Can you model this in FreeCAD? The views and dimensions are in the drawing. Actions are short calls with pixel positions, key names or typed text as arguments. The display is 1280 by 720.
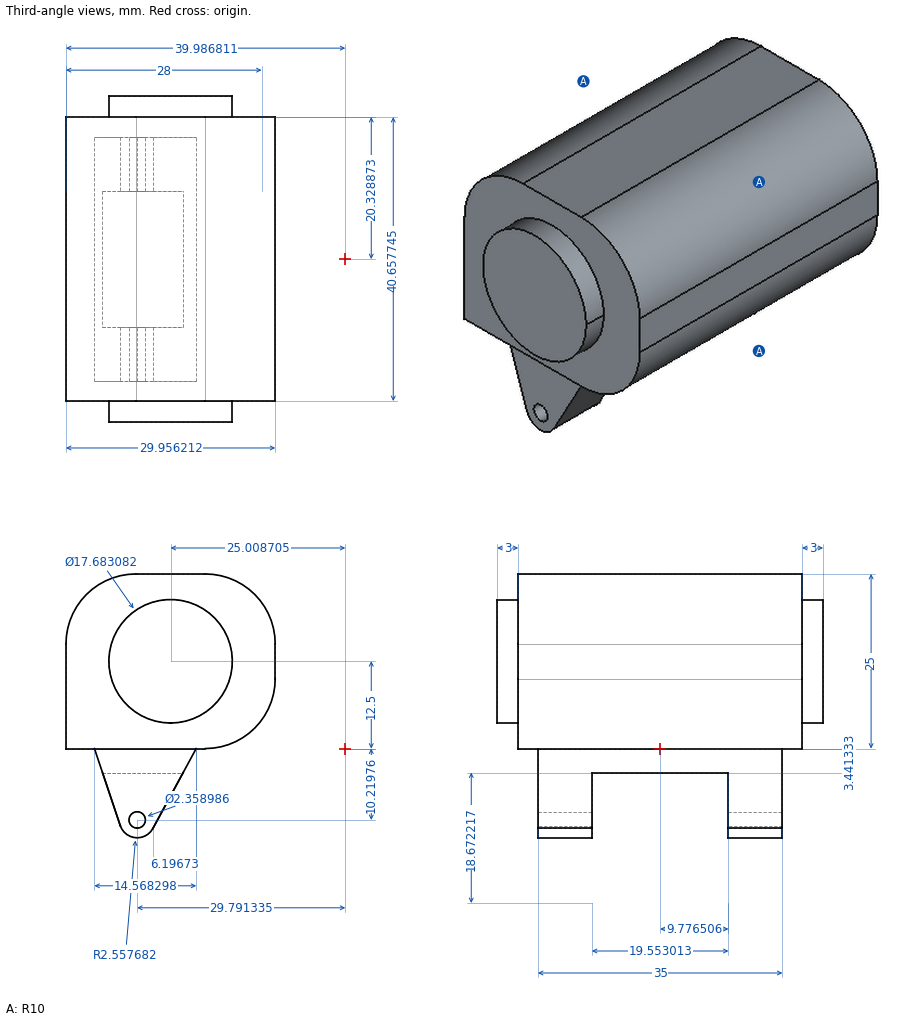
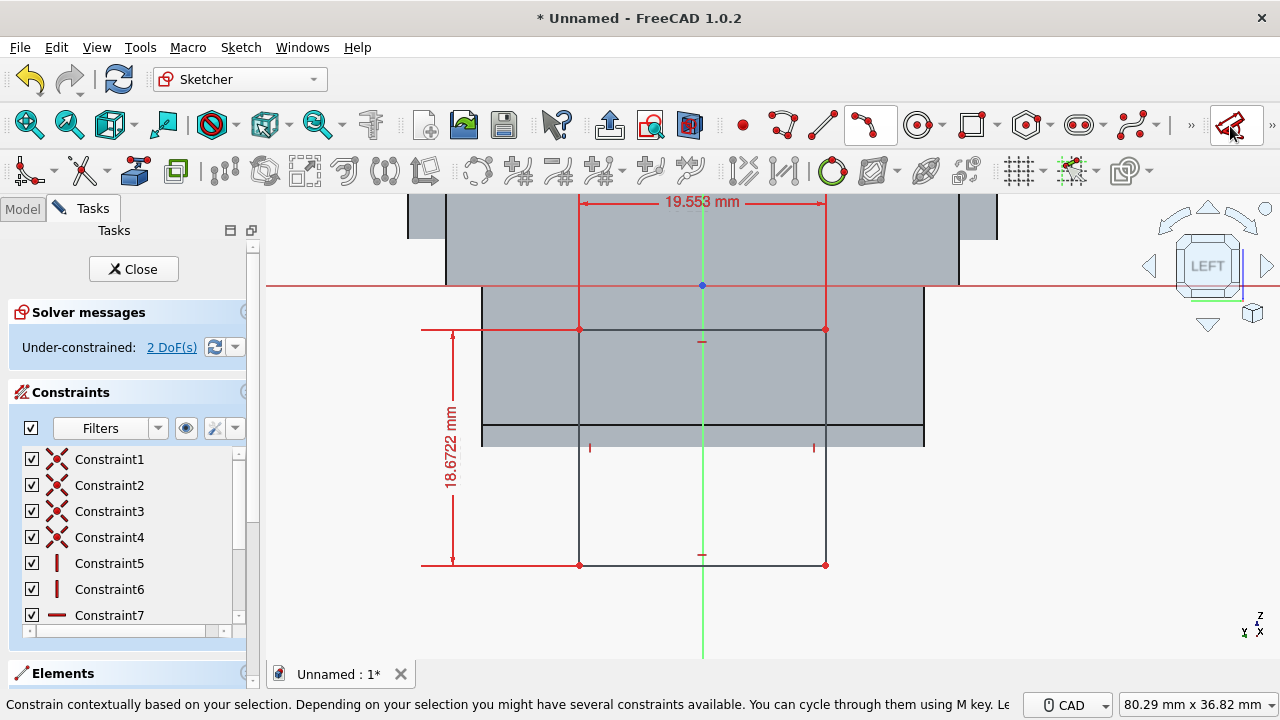
click(579, 330)
click(641, 252)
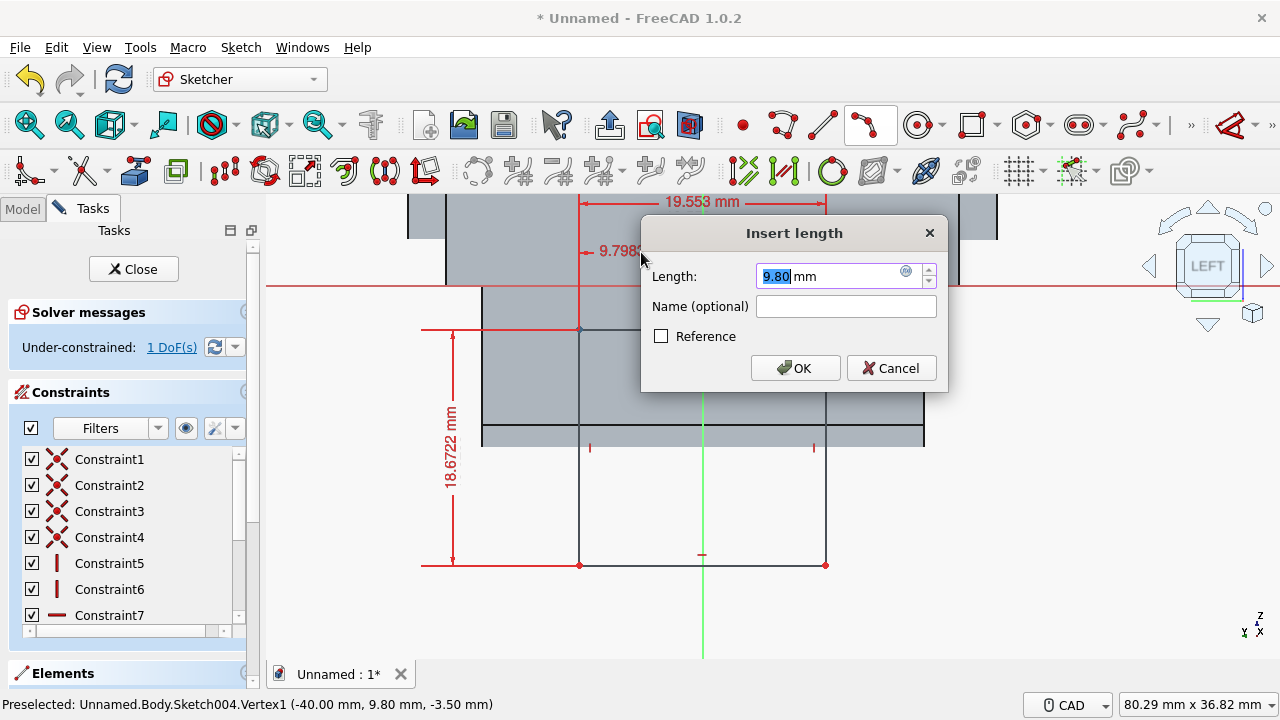
text(9.776506)
key(Return)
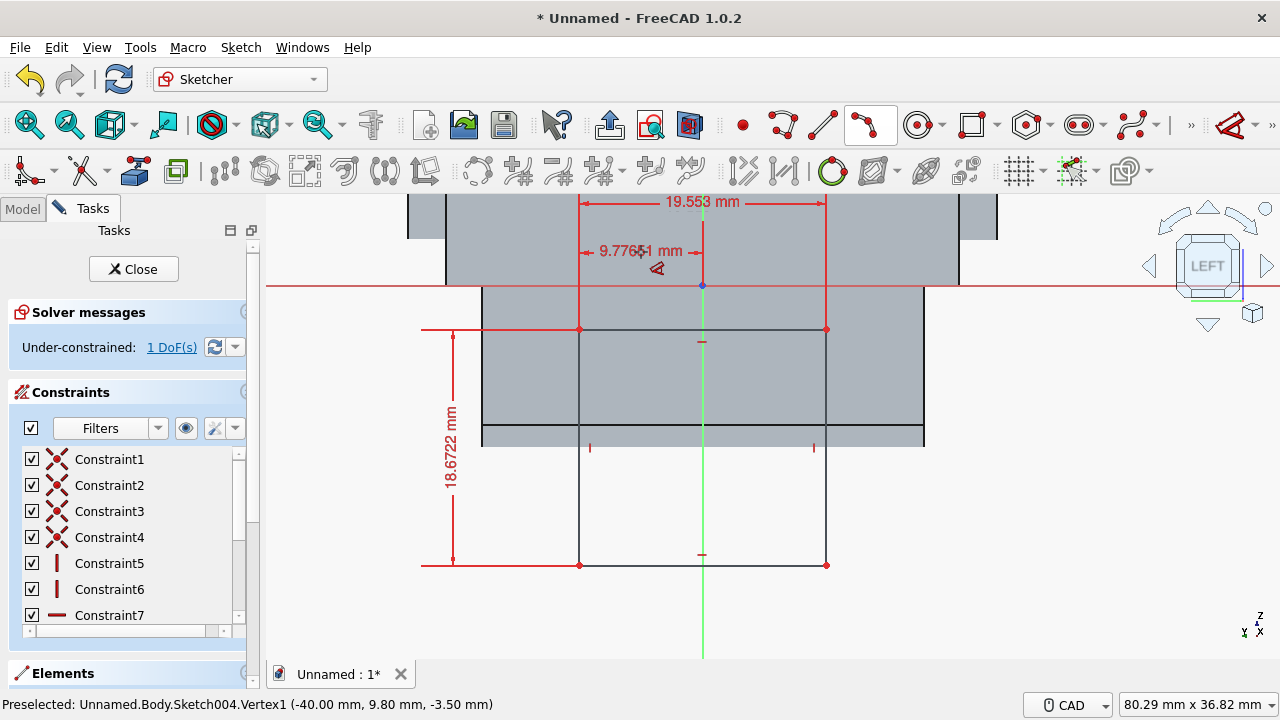
click(579, 330)
click(545, 308)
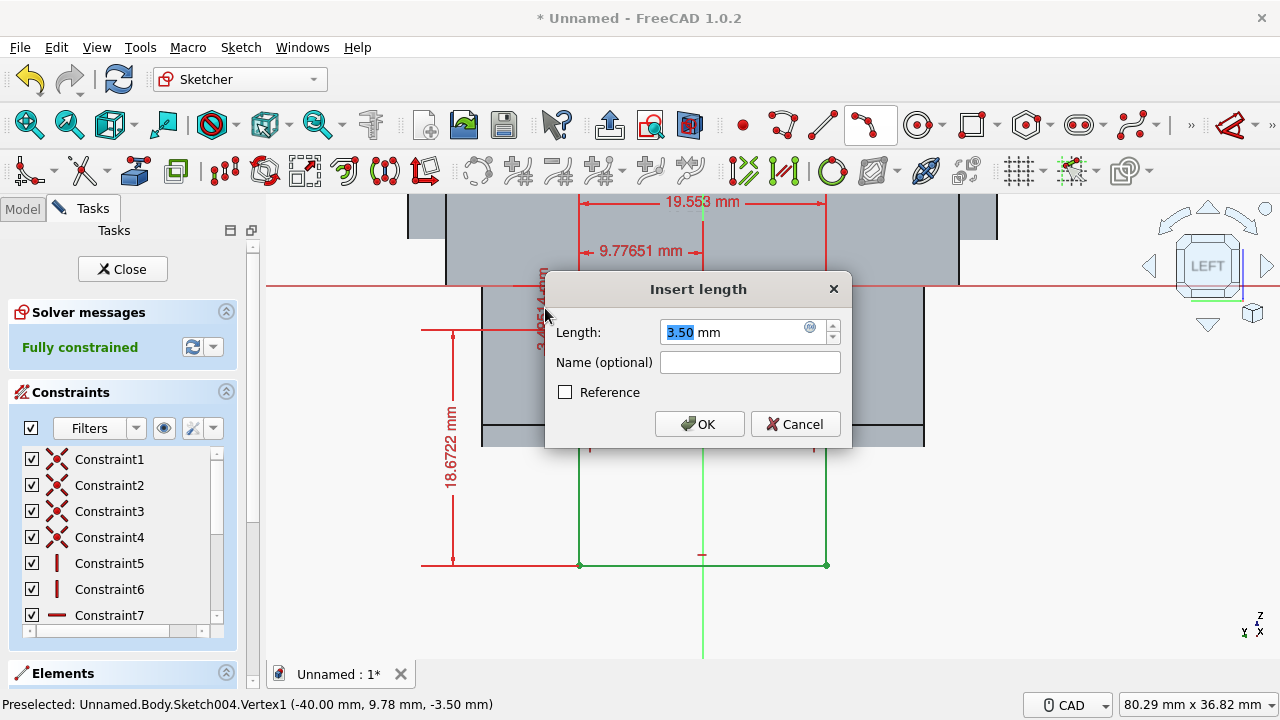
text(3.441333)
key(Return)
key(Escape)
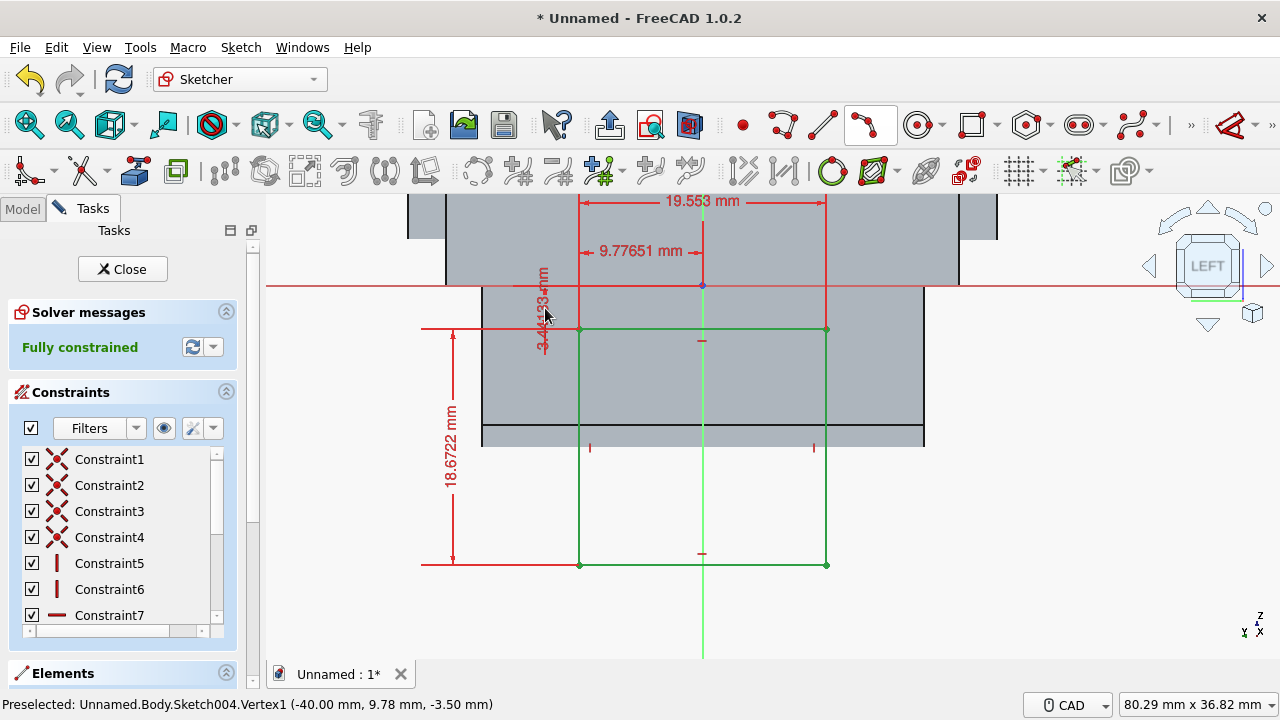
click(123, 269)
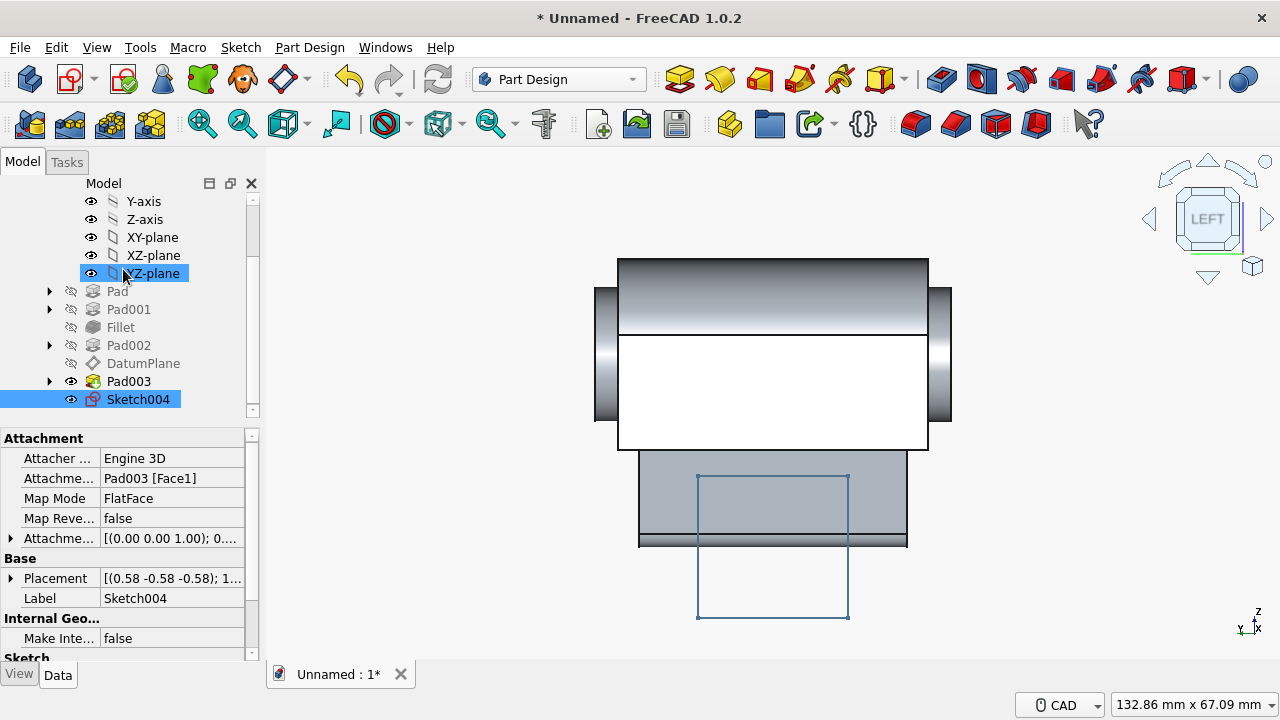
click(942, 80)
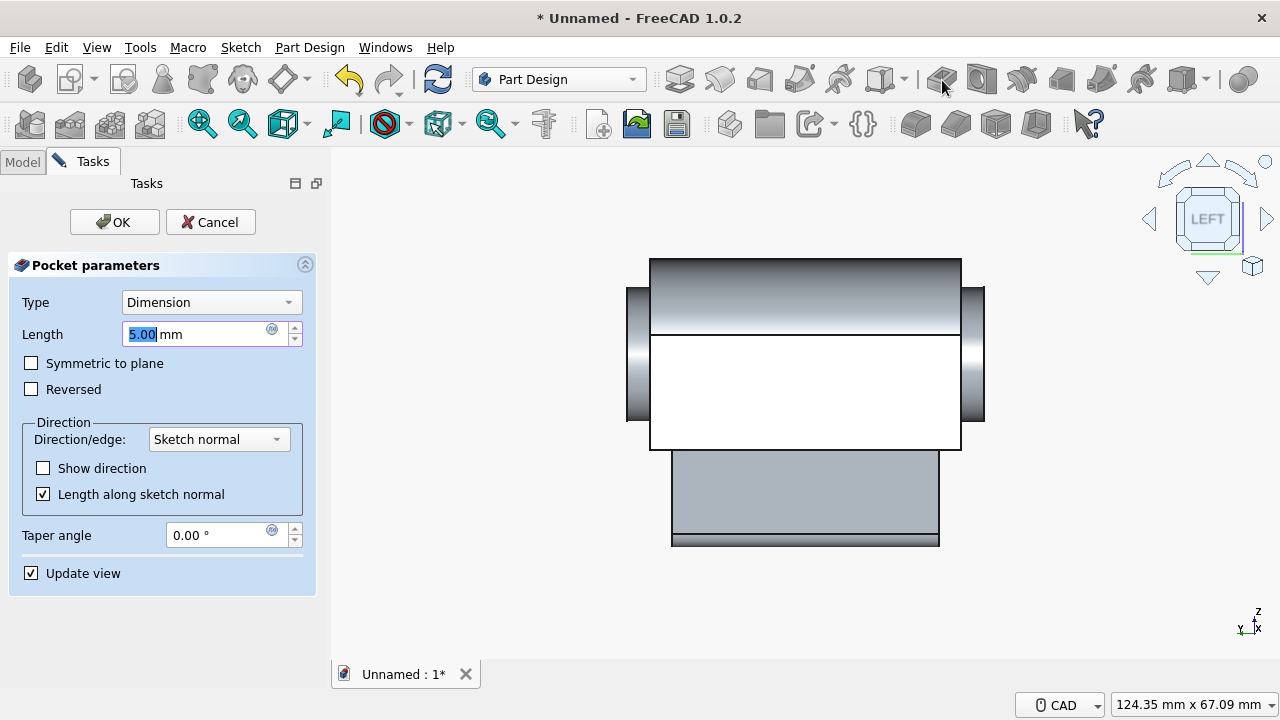
text(28)
key(Tab)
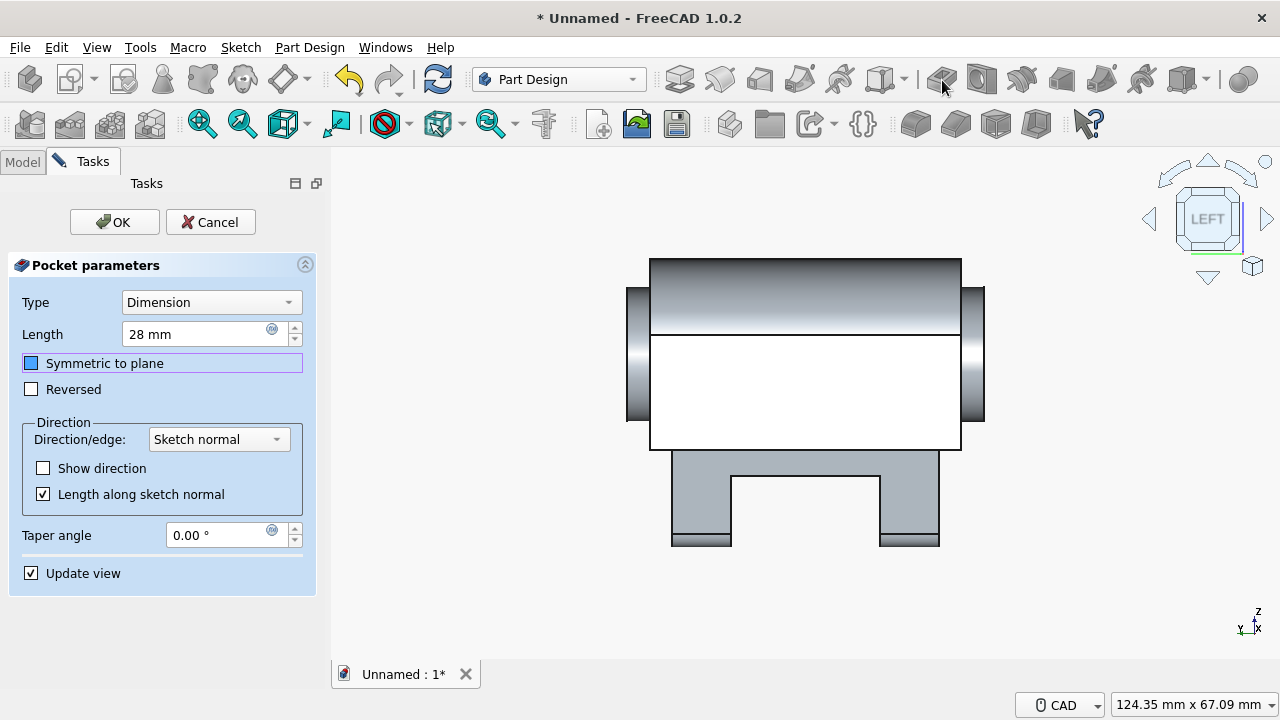
click(115, 222)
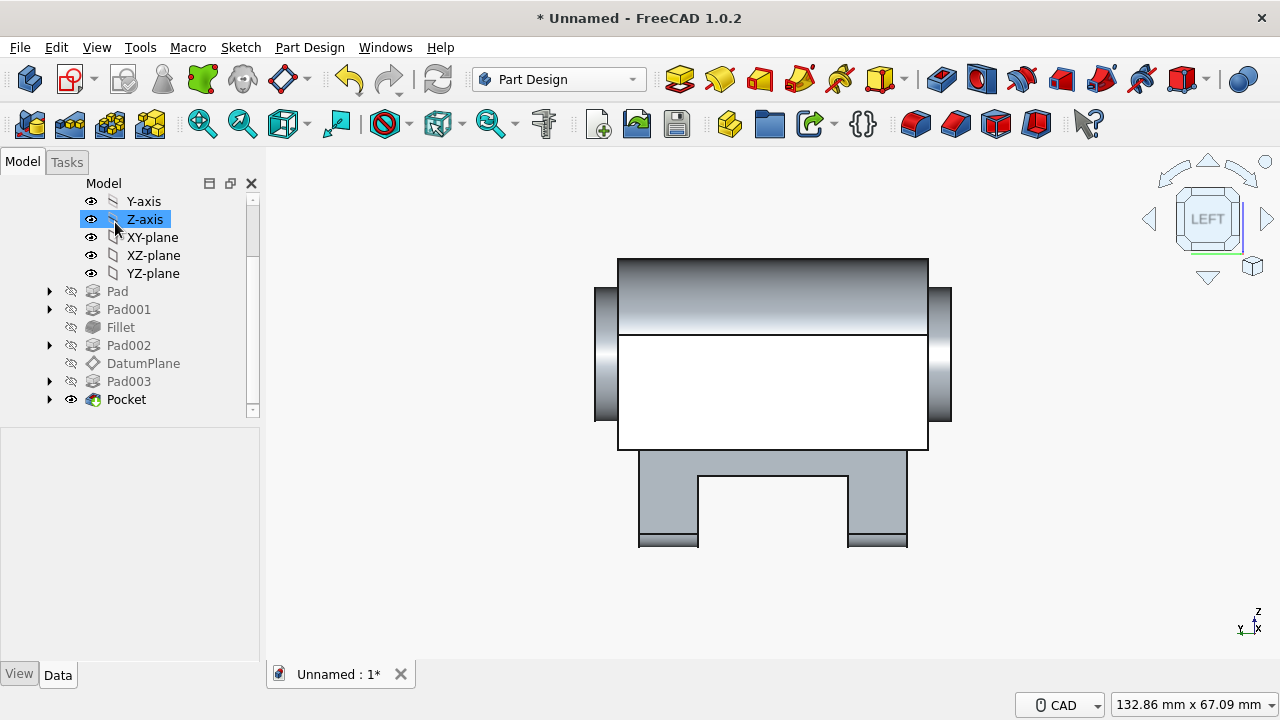
key(0)